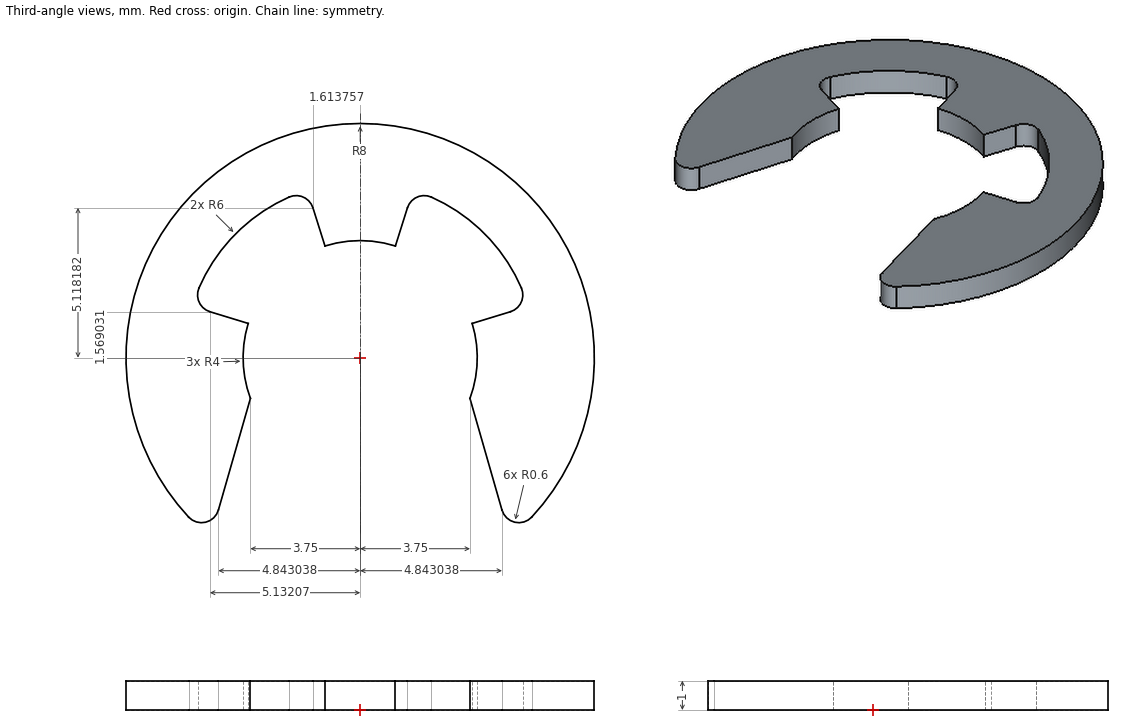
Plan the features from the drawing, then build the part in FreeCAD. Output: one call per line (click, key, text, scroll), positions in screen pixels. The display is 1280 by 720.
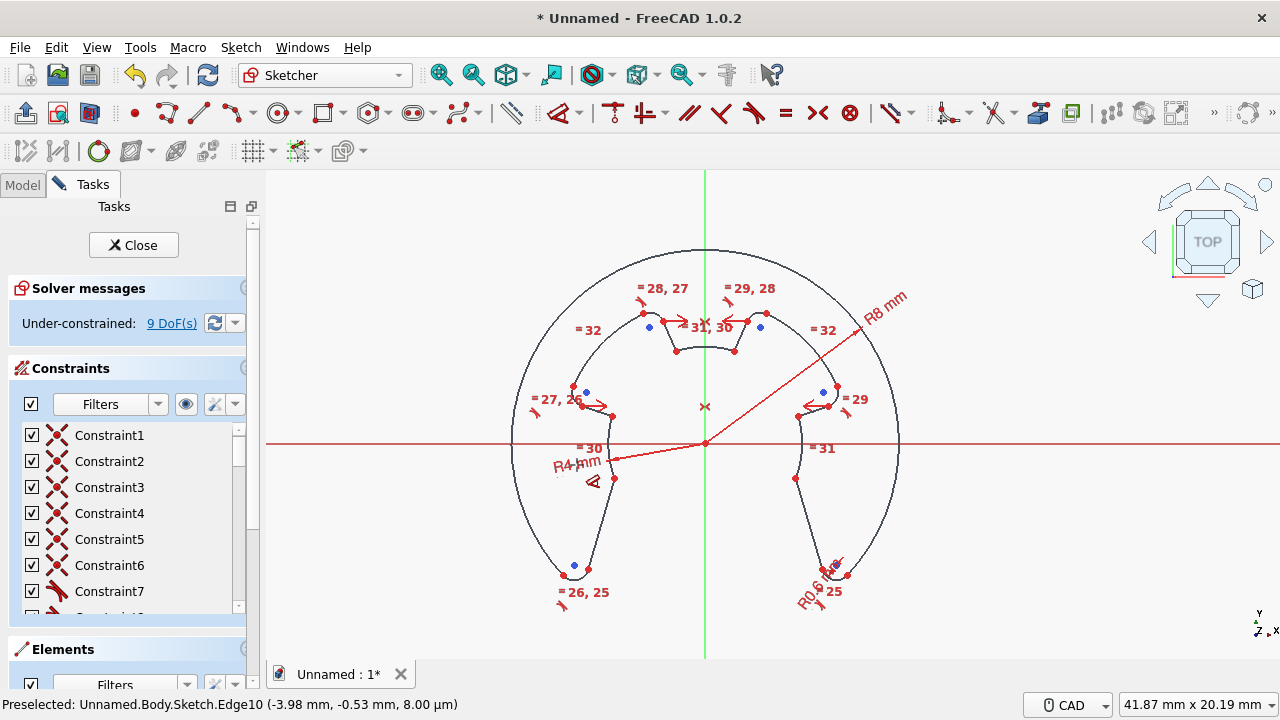
click(617, 330)
click(597, 305)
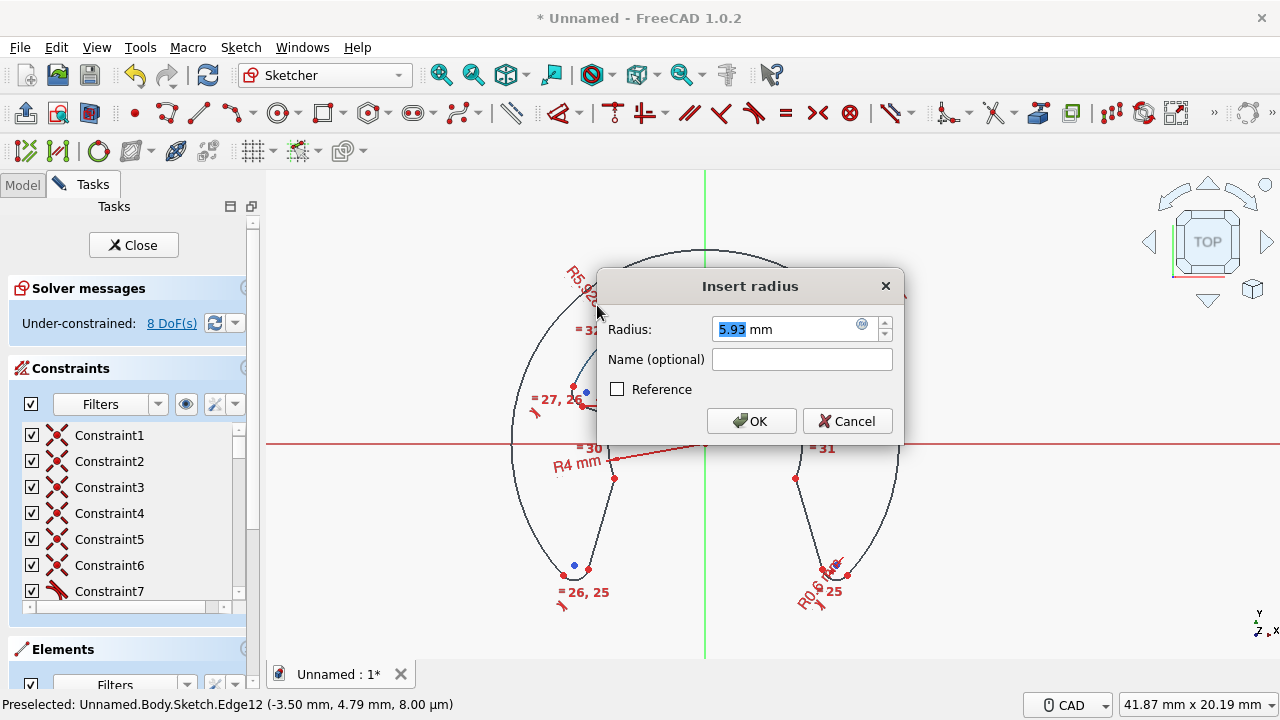
text(6)
key(Return)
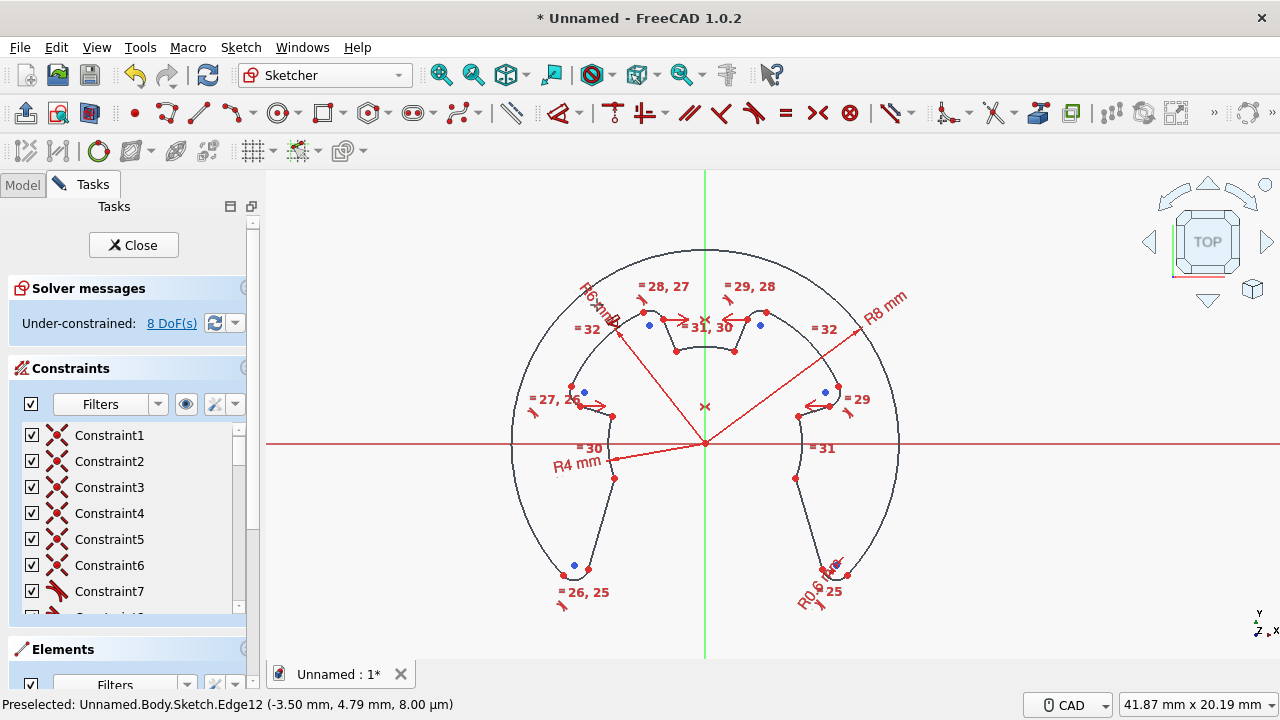
click(796, 478)
click(750, 512)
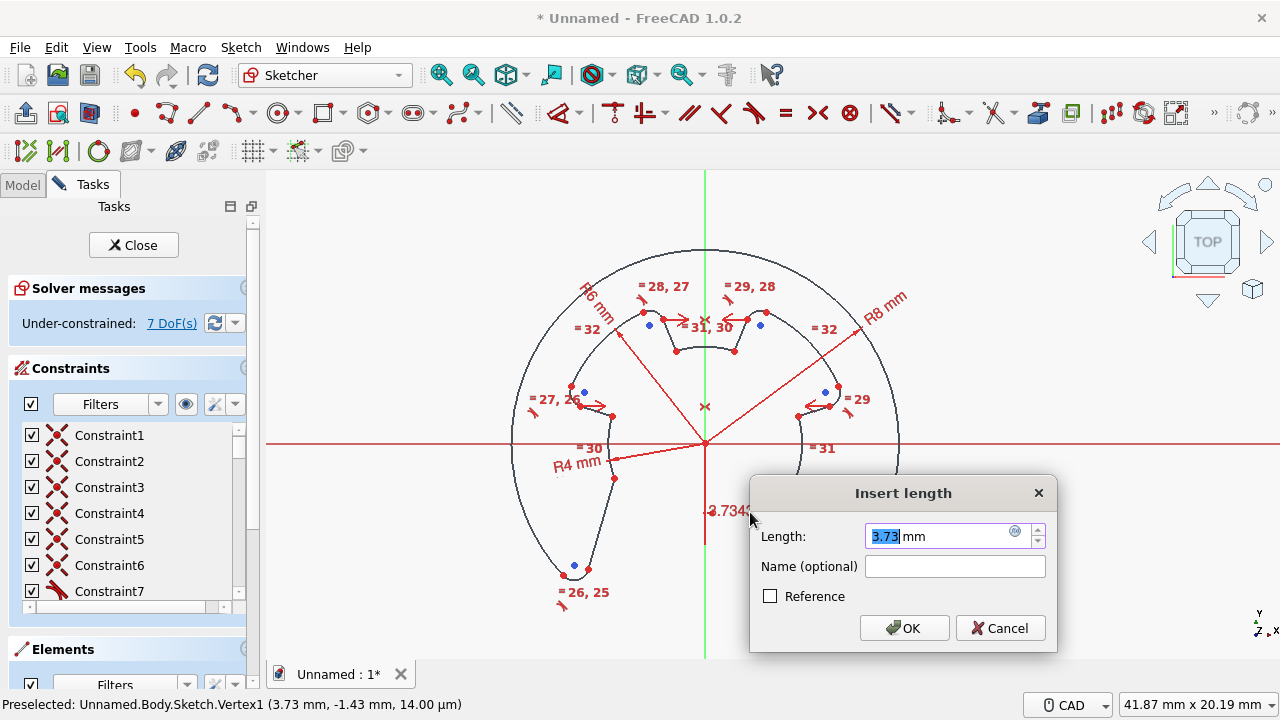
text(3.75)
key(Return)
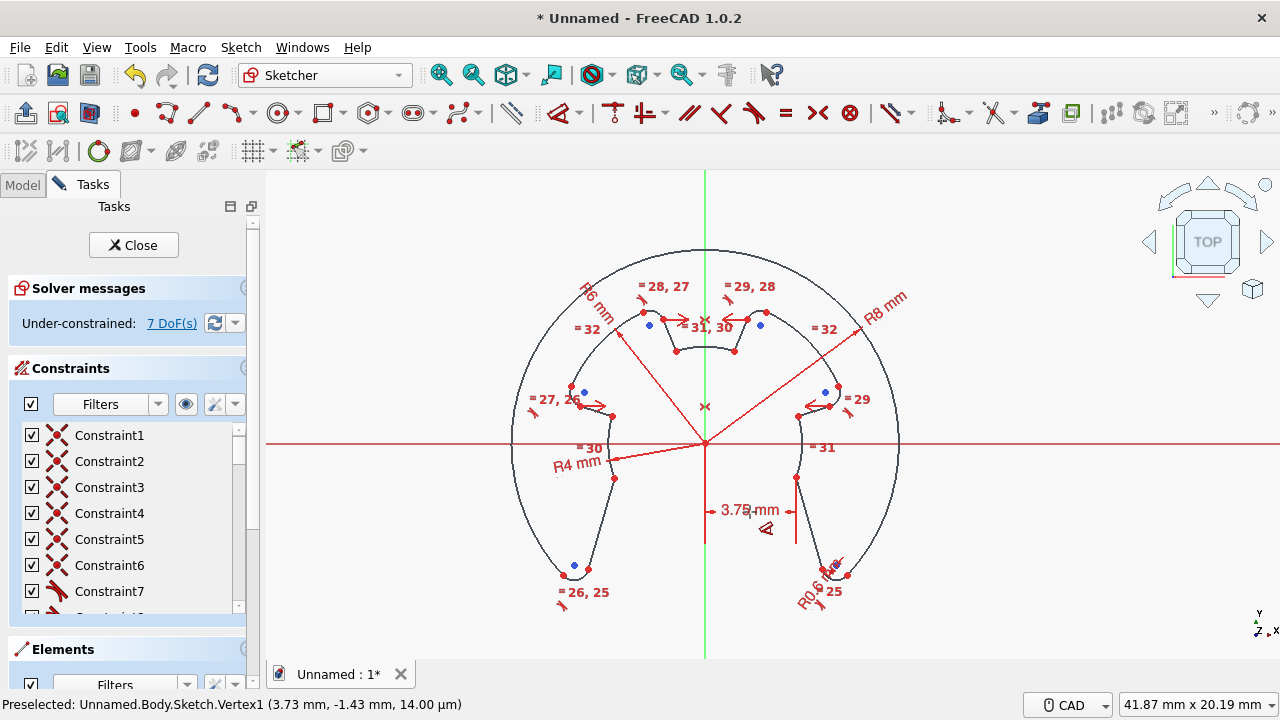
click(615, 478)
click(660, 512)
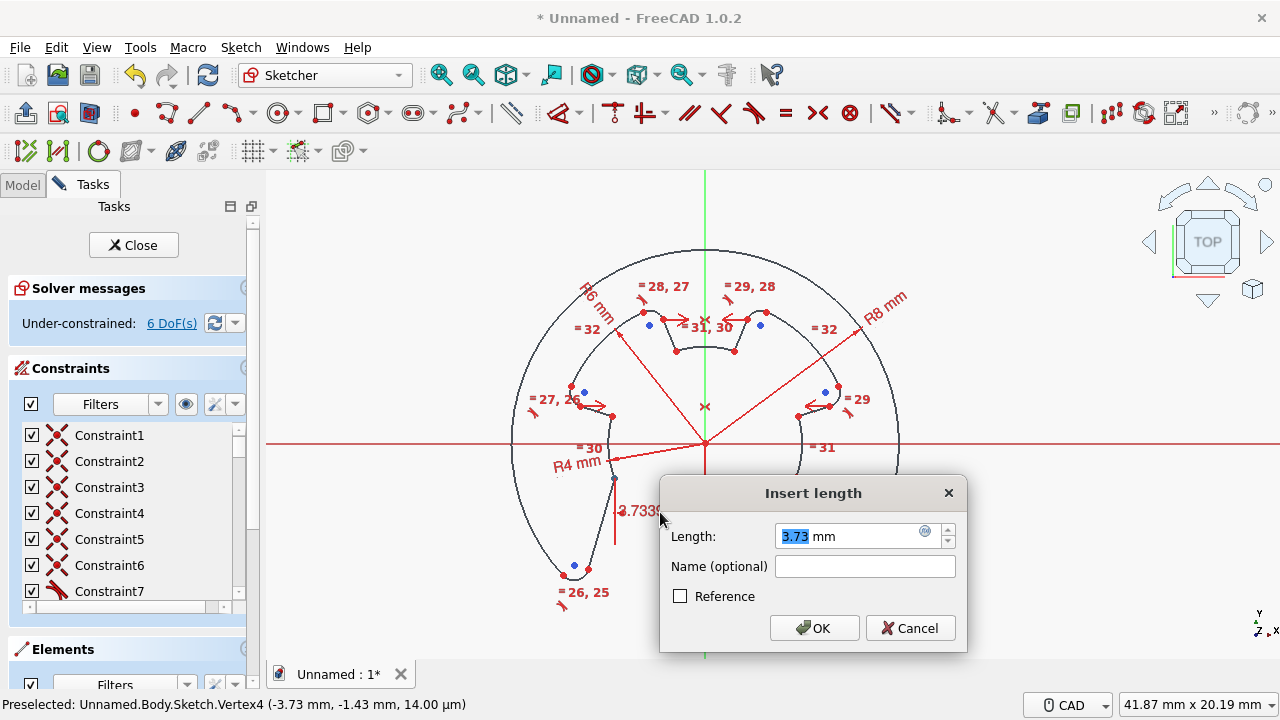
text(3.75)
key(Return)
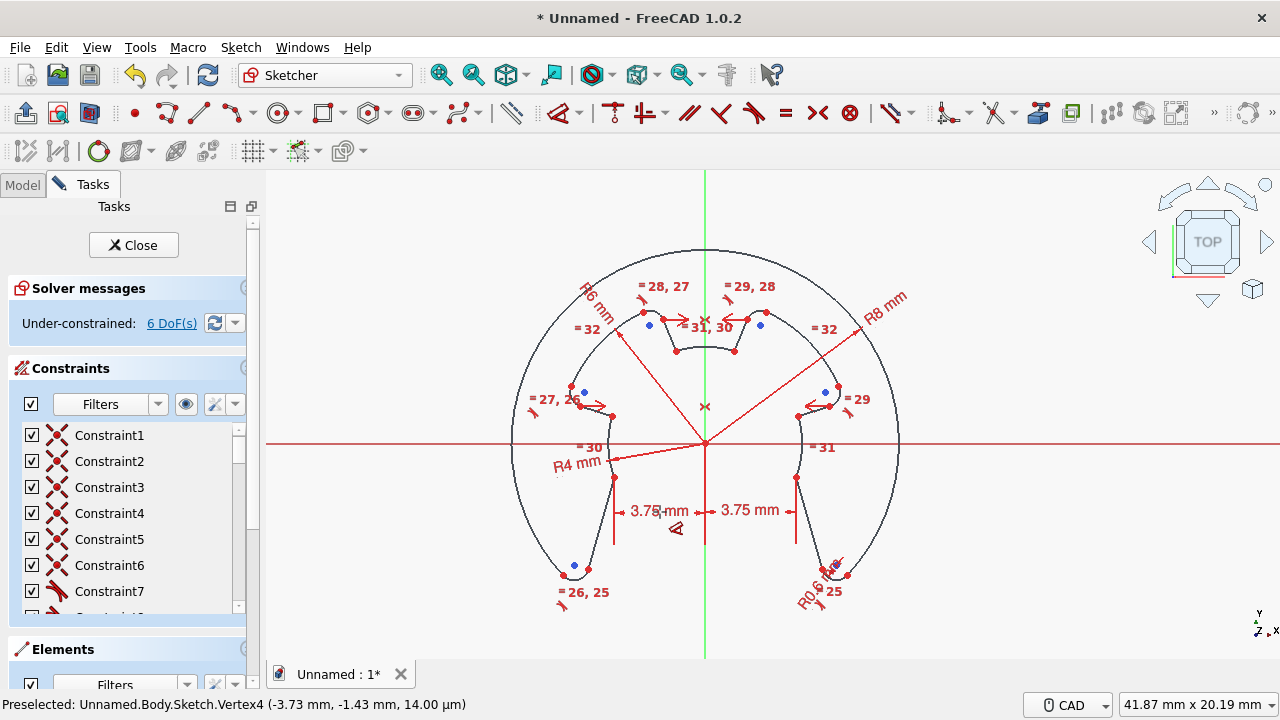
click(580, 406)
click(672, 478)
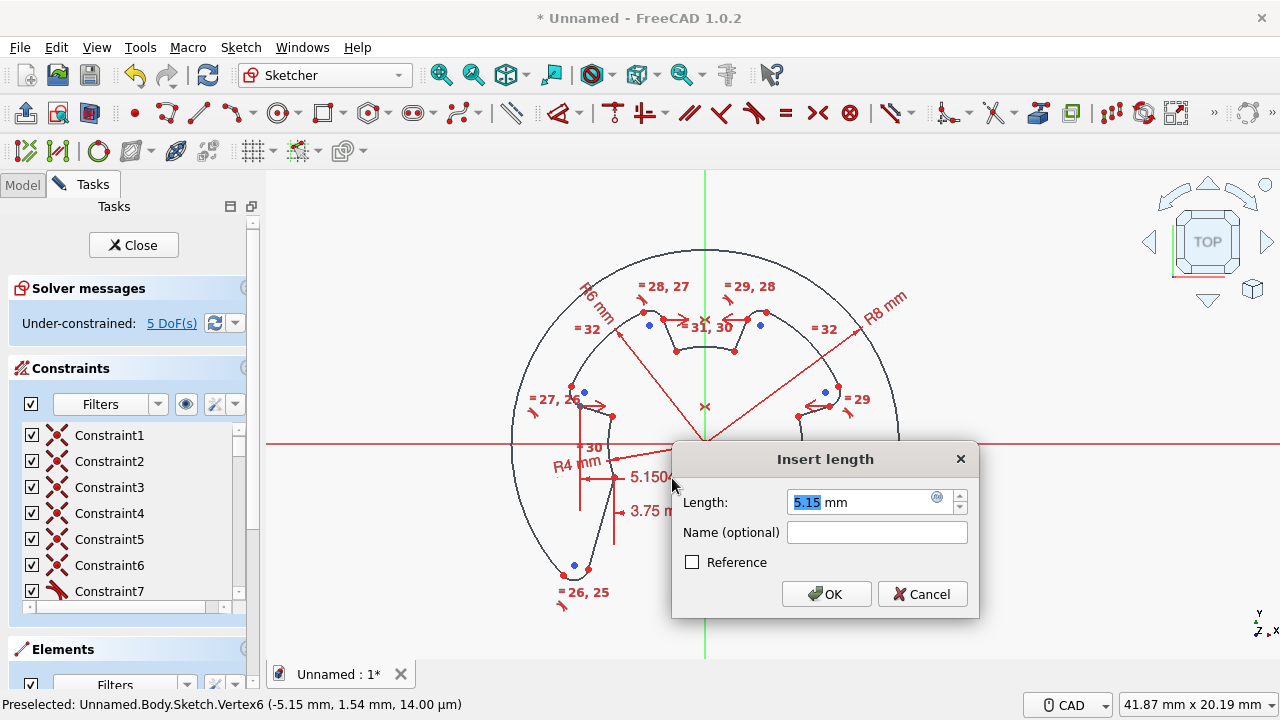
text(5.13207)
key(Return)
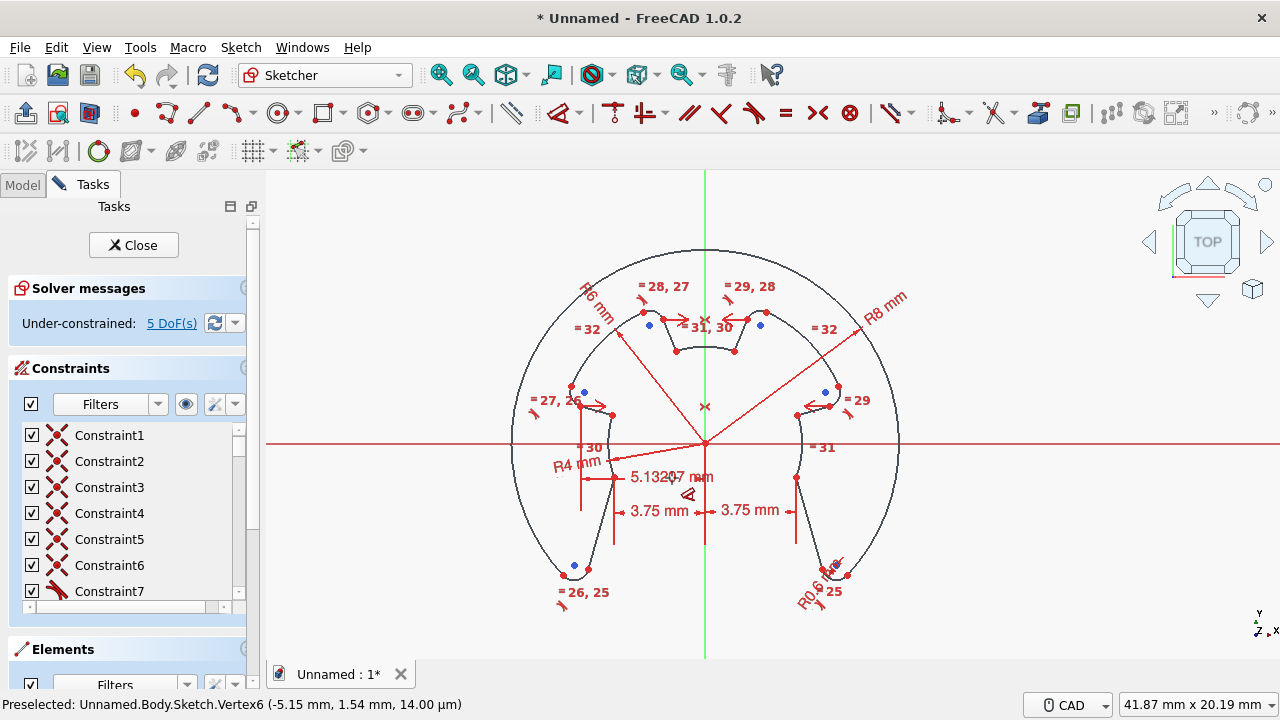
click(823, 570)
click(737, 604)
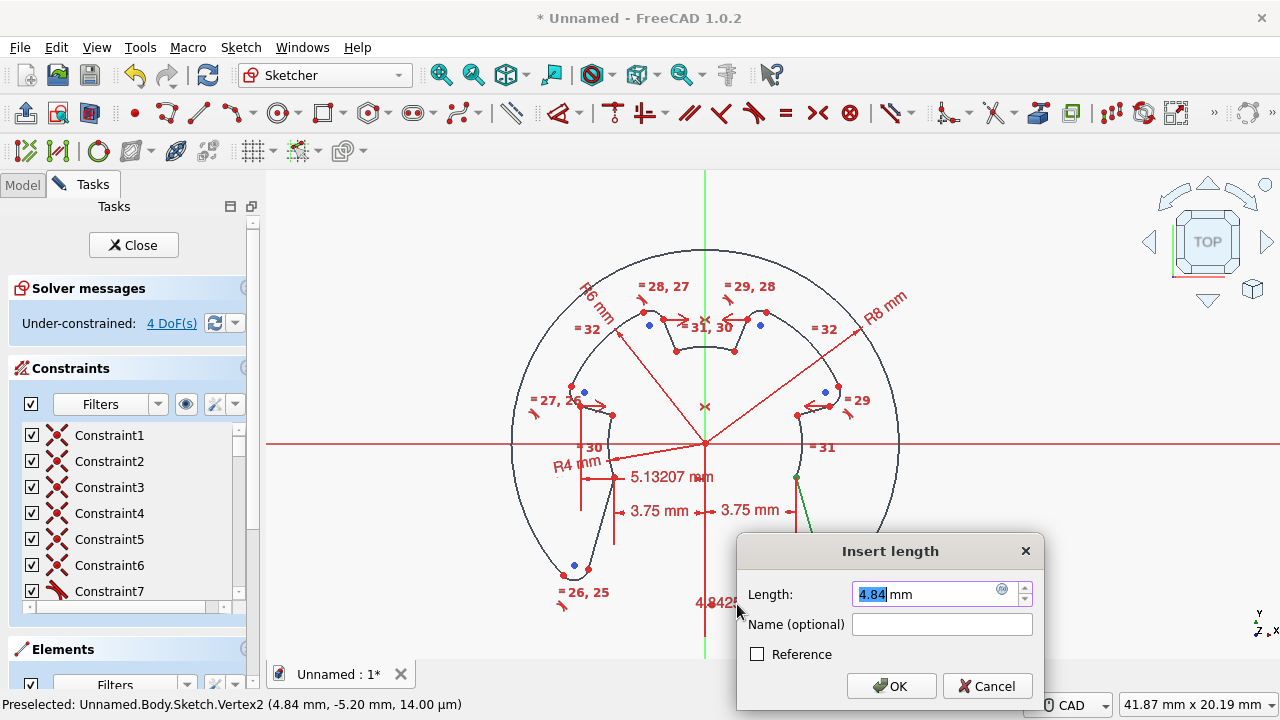
text(4.843038)
key(Return)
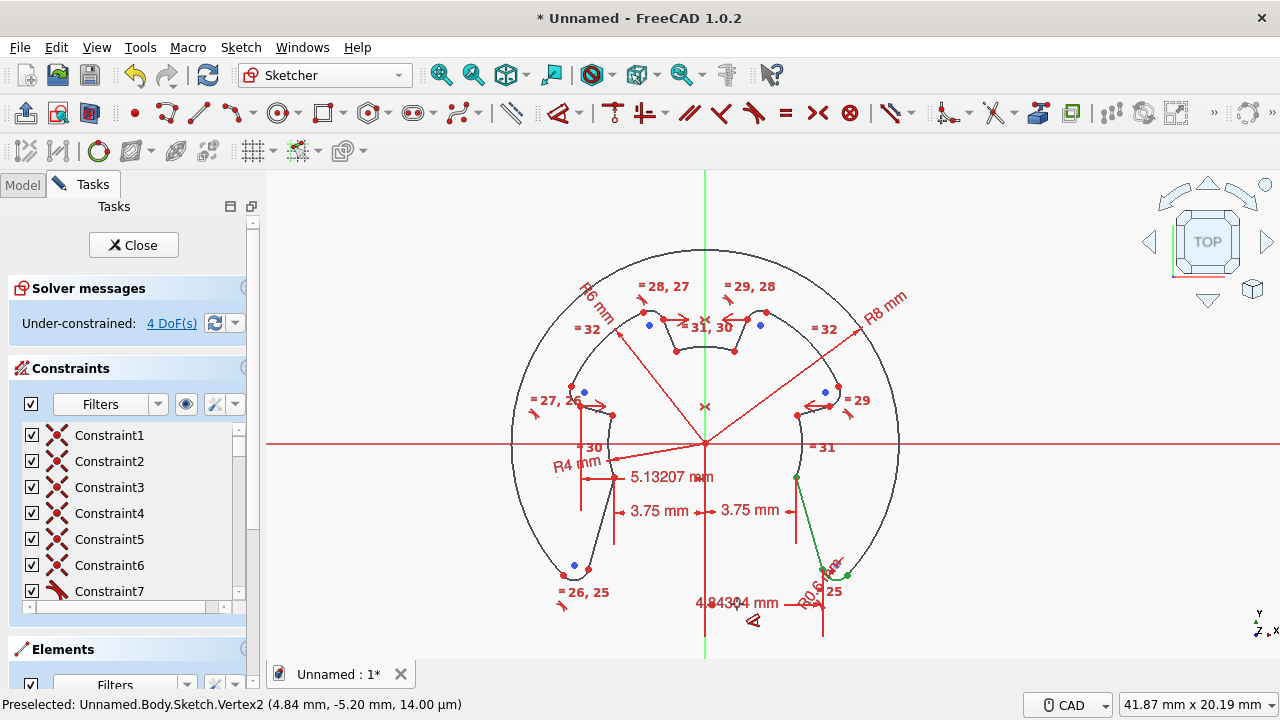
click(588, 570)
click(647, 604)